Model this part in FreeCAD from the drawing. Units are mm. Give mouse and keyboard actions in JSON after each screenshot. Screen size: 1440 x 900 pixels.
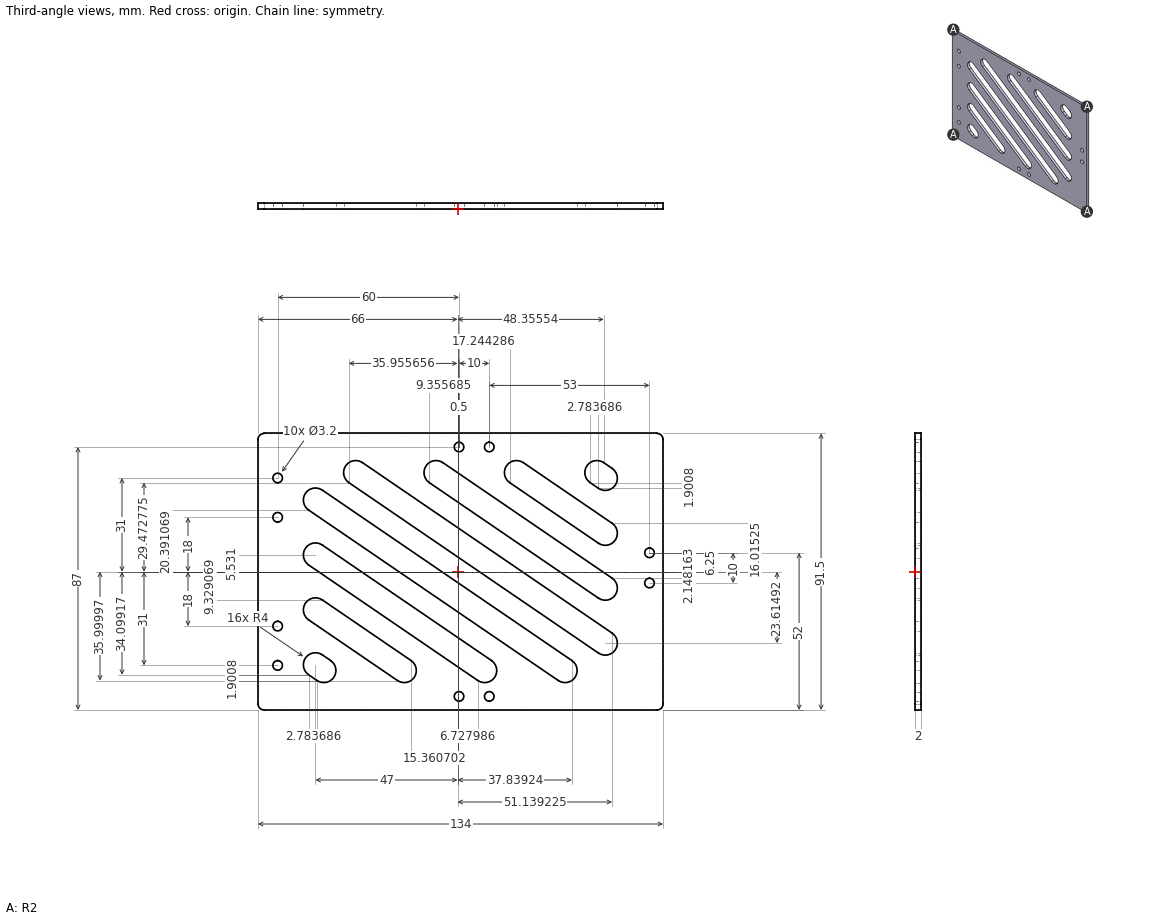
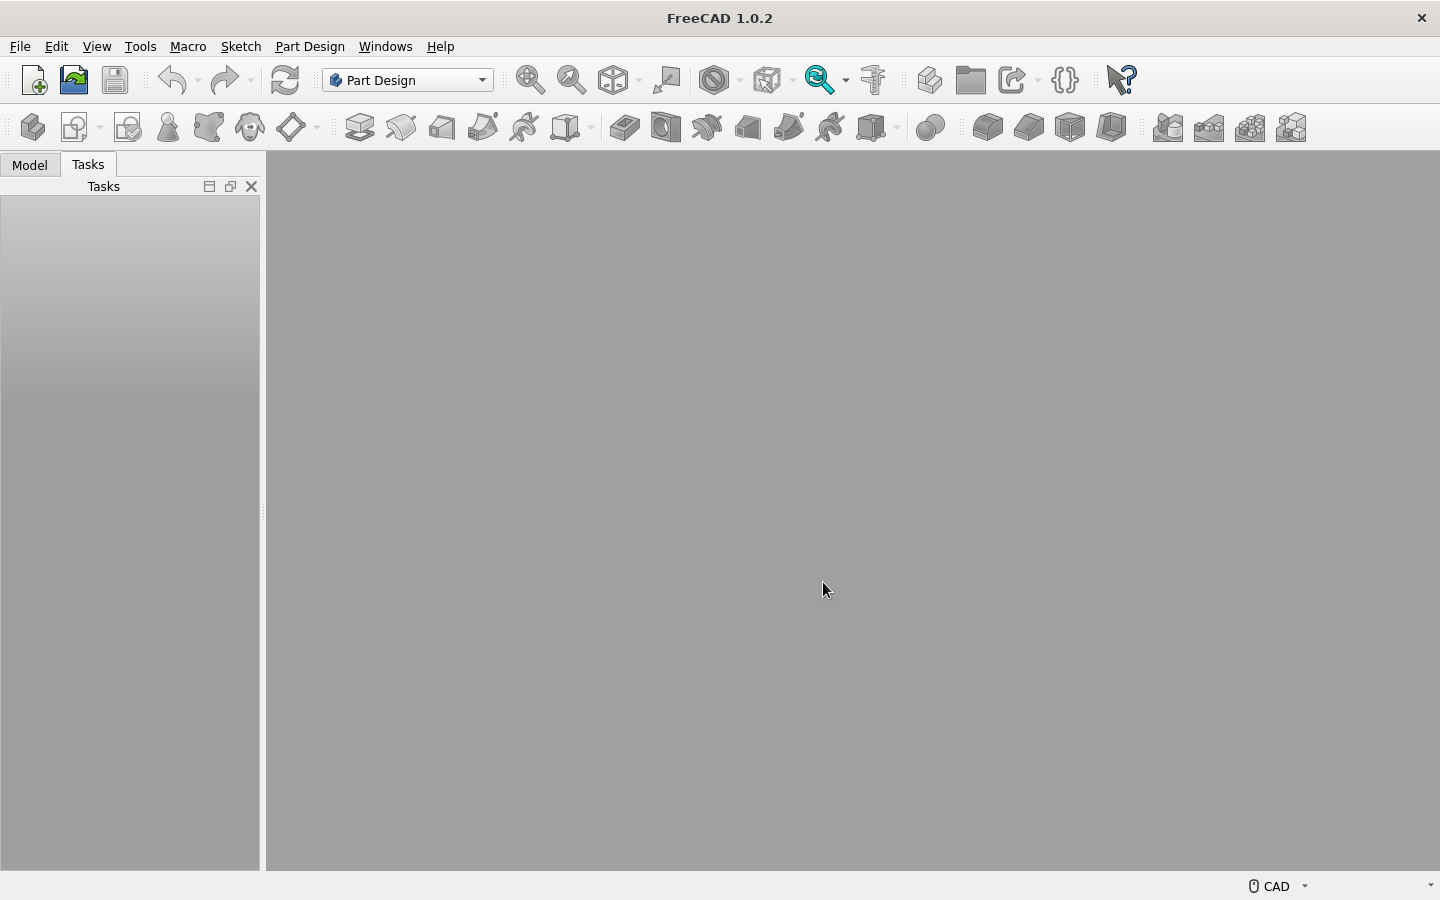
{"action": "left_click", "coordinate": [33, 80]}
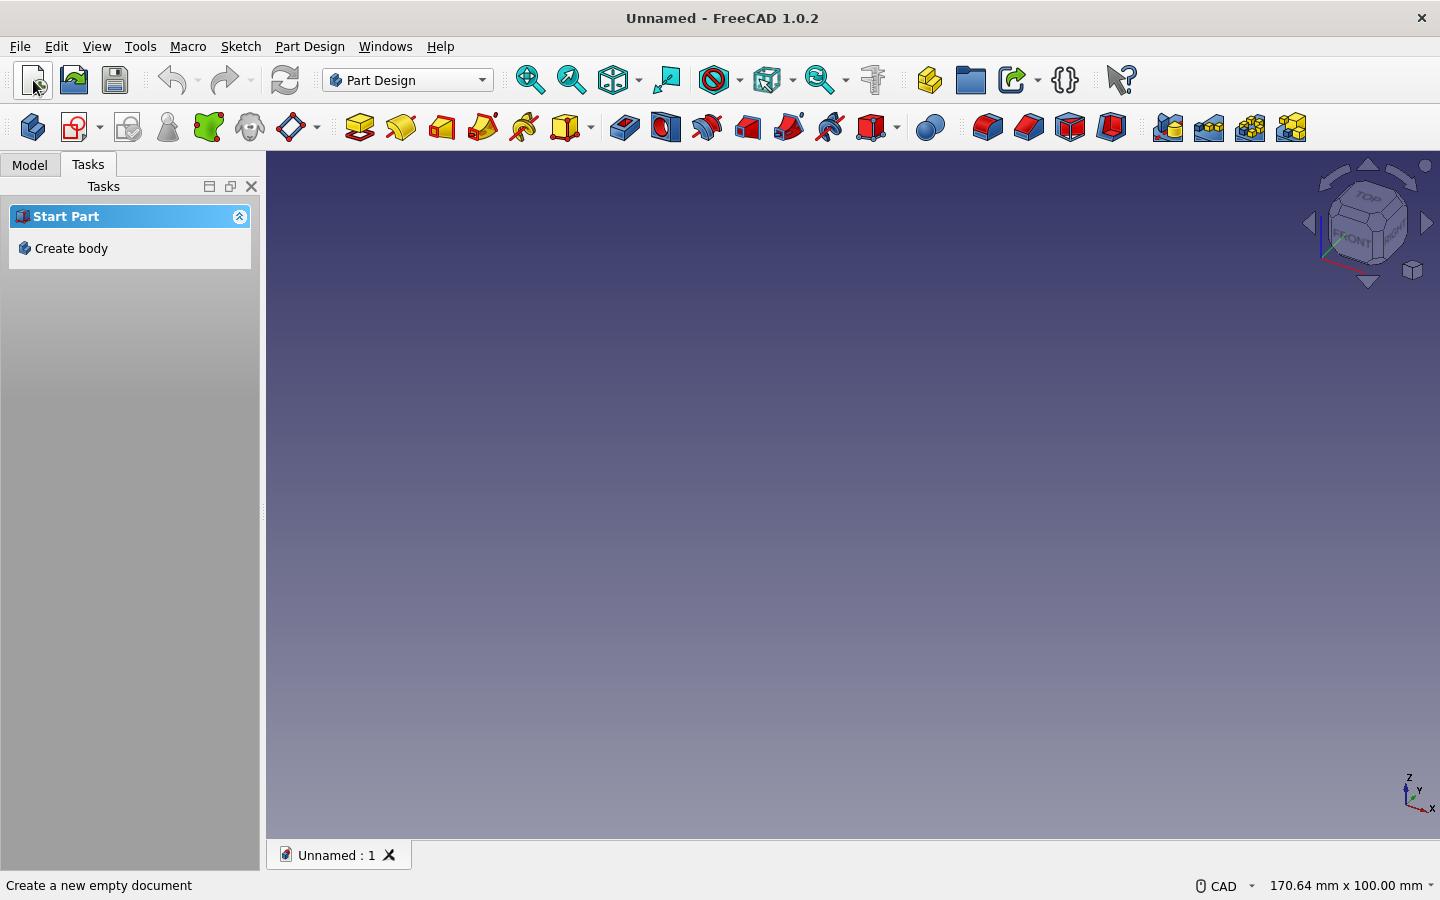
{"action": "left_click", "coordinate": [74, 128]}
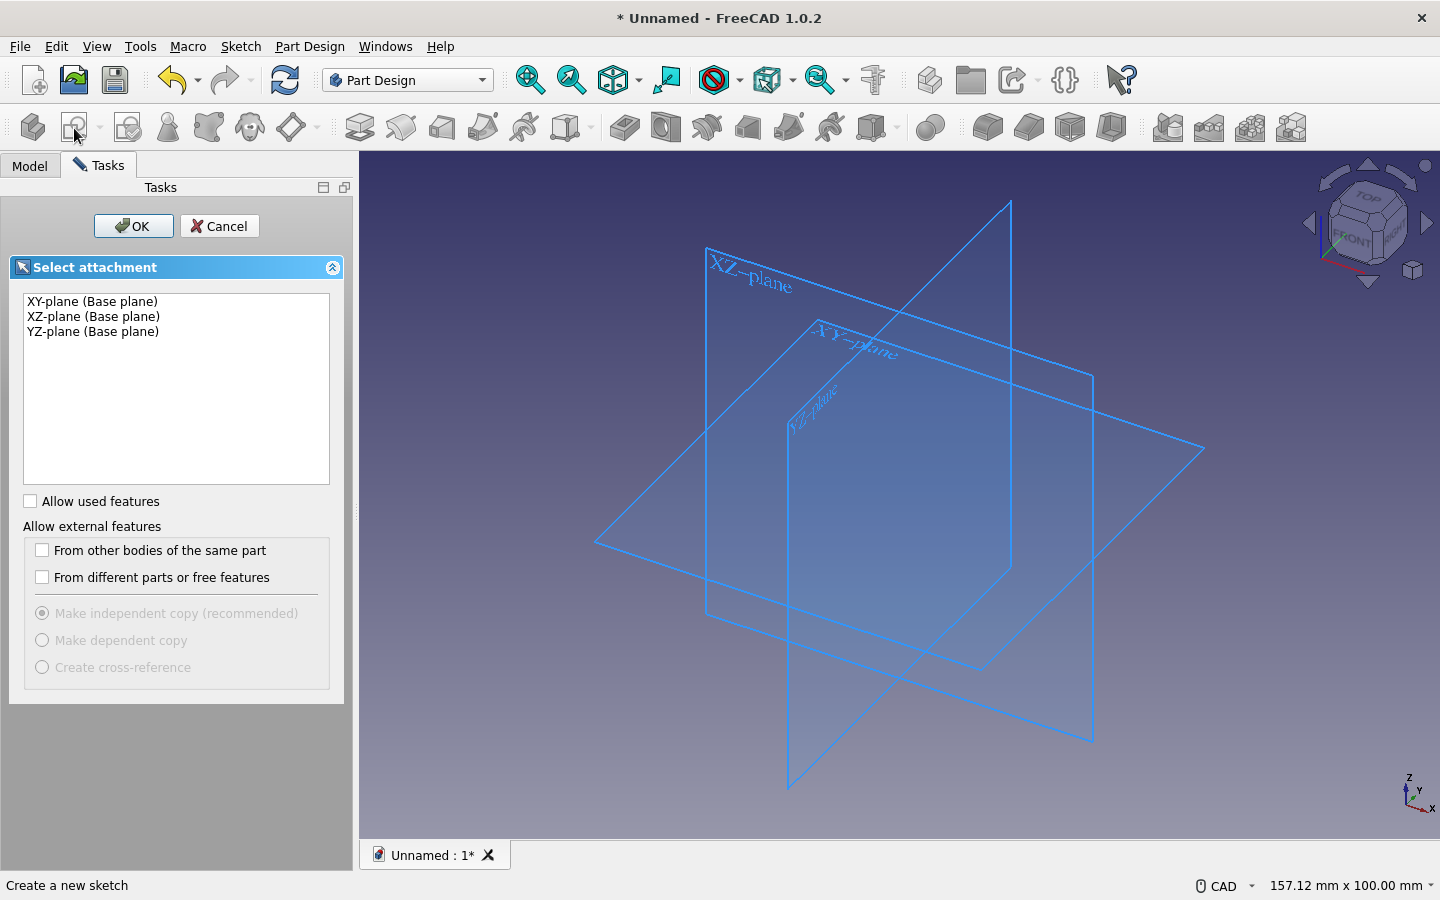
{"action": "left_click", "coordinate": [84, 316]}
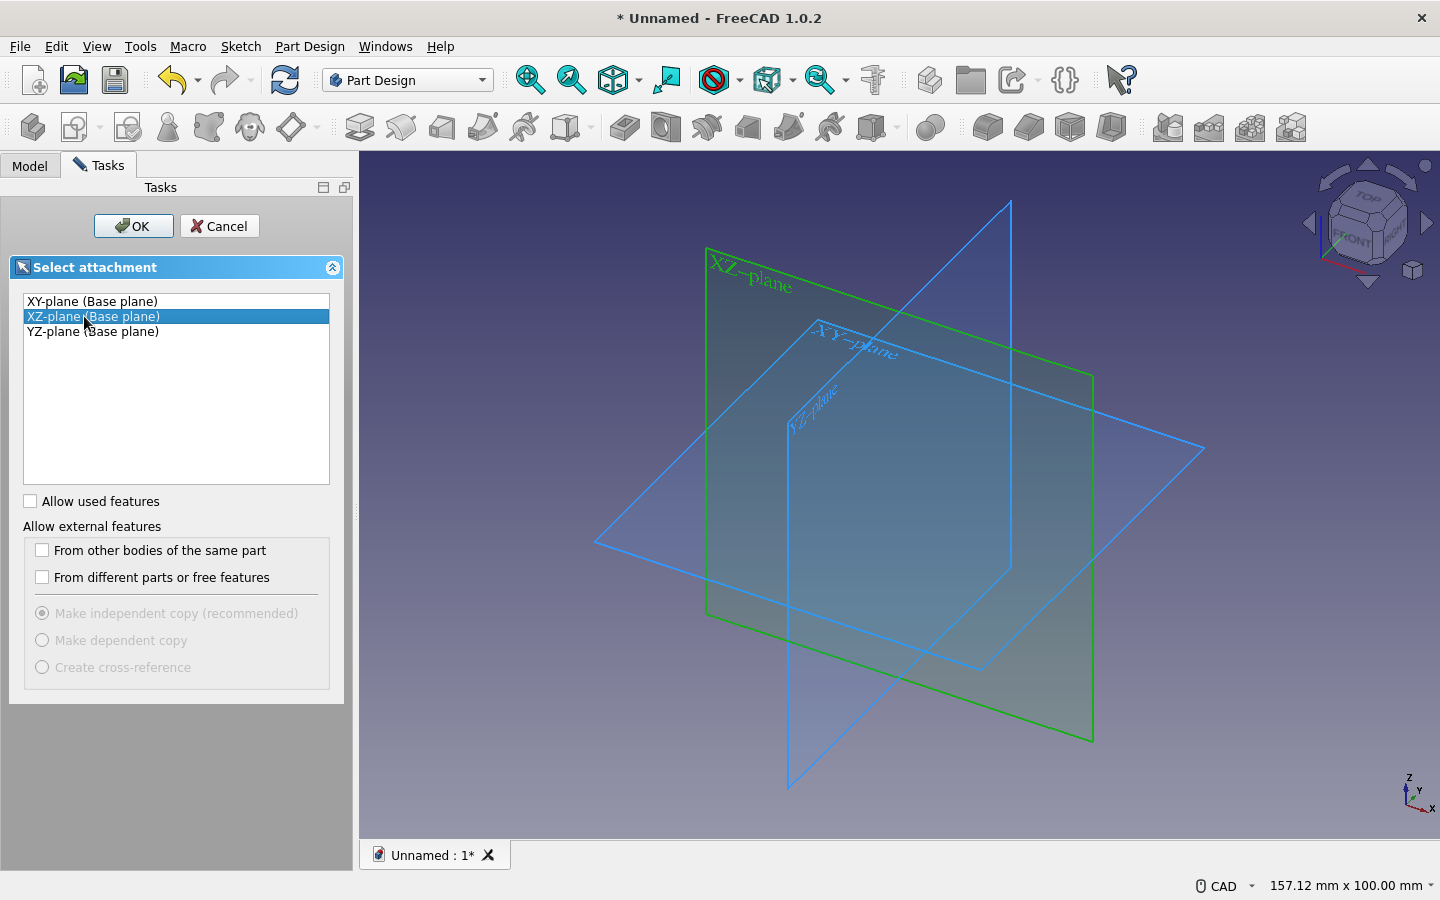
{"action": "left_click", "coordinate": [134, 226]}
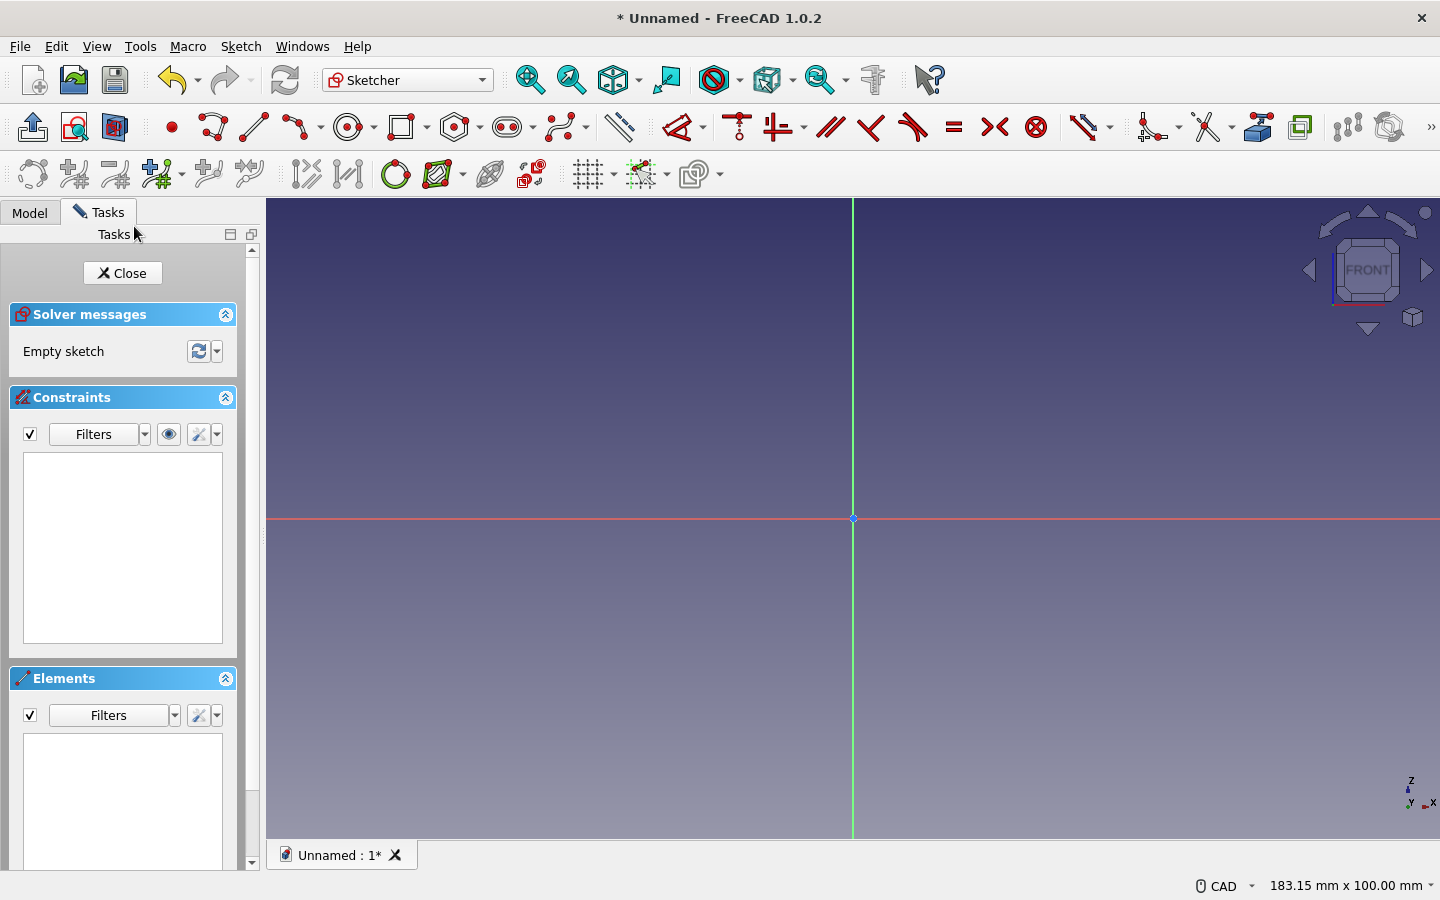
{"action": "scroll", "coordinate": [632, 518], "scroll_direction": "down", "scroll_amount": 2}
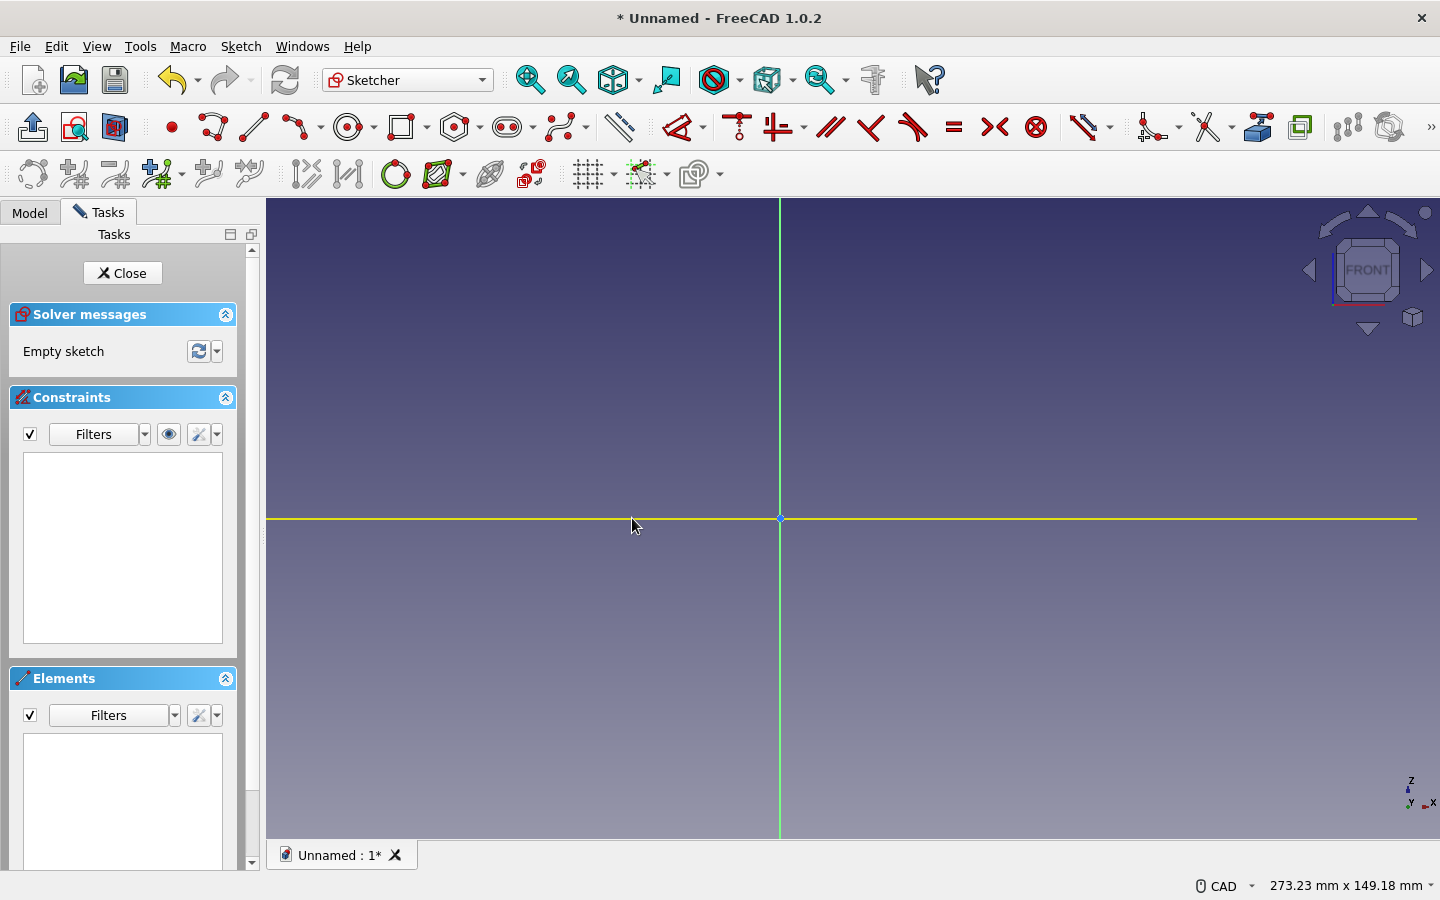
{"action": "left_click", "coordinate": [400, 128]}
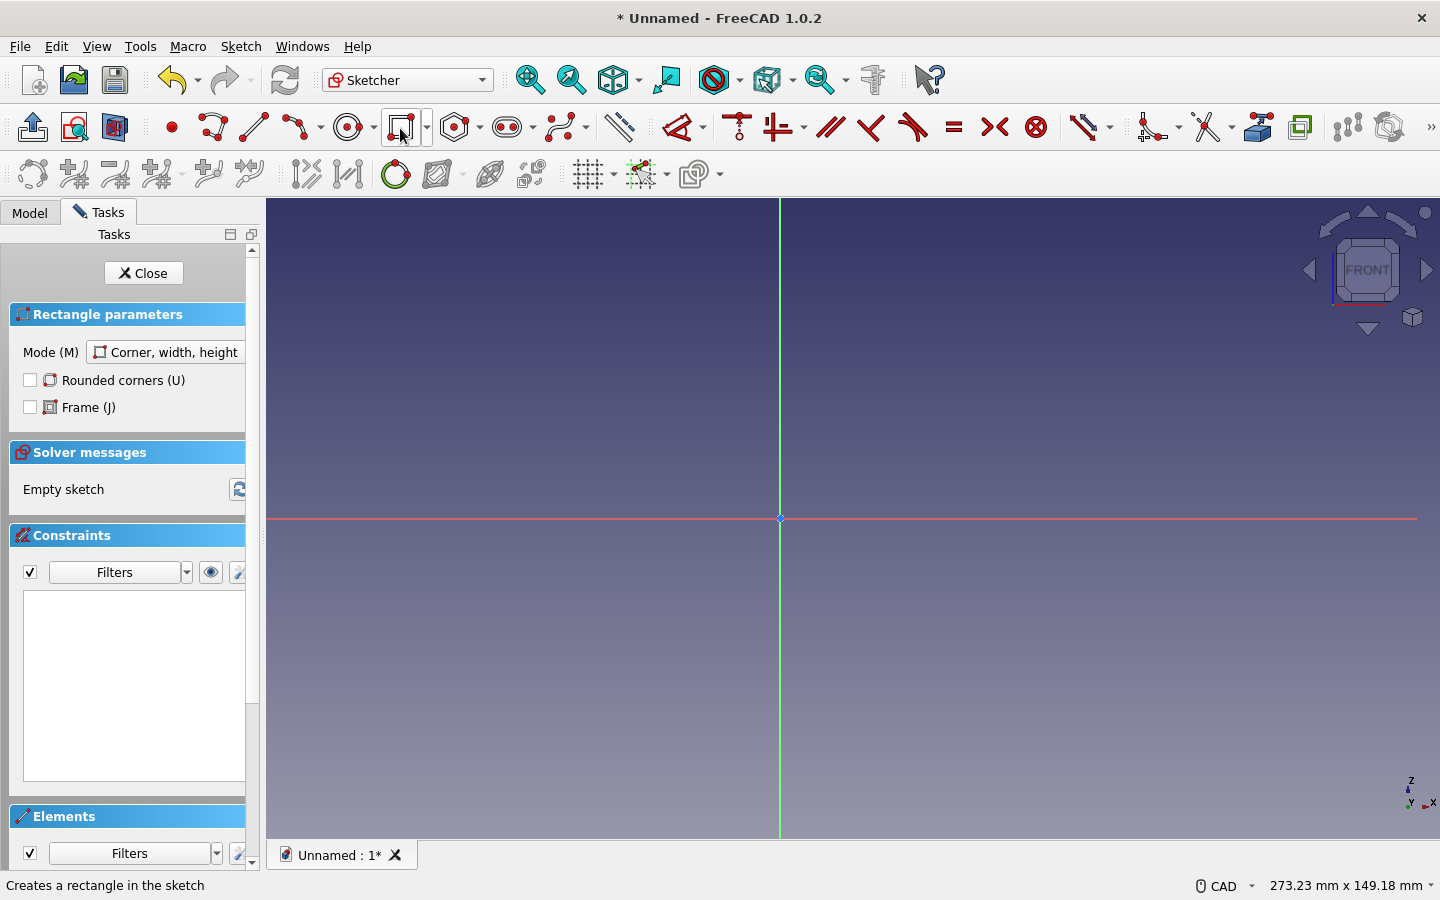
{"action": "left_click", "coordinate": [497, 322]}
{"action": "mouse_move", "coordinate": [1072, 715]}